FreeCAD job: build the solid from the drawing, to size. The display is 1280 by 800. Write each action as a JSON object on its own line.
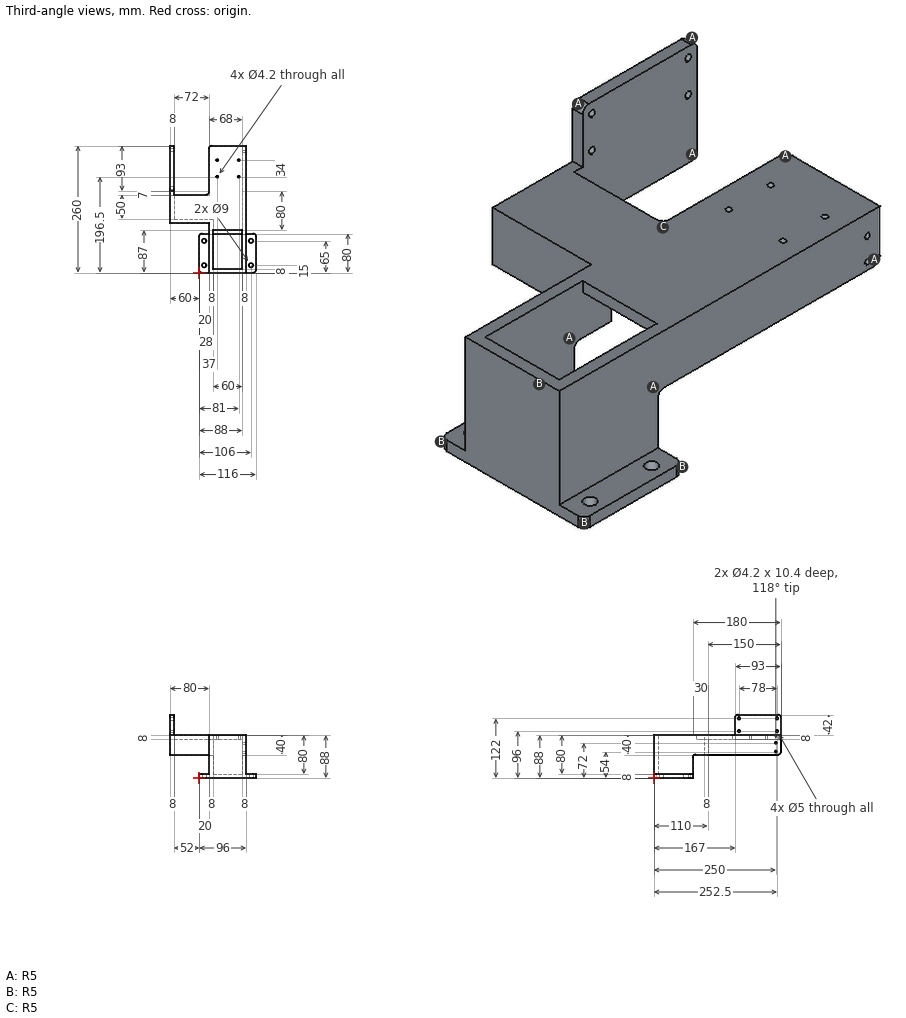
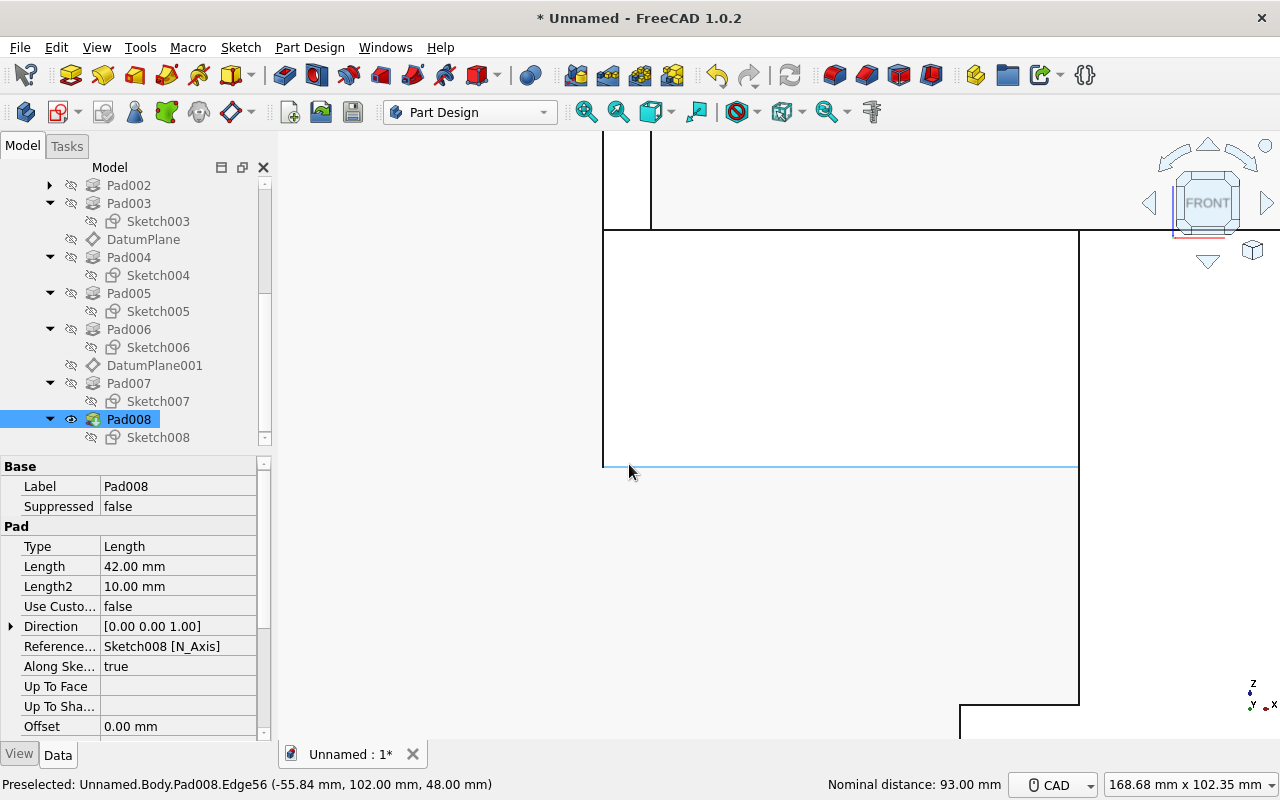
{"action": "left_click", "coordinate": [588, 112]}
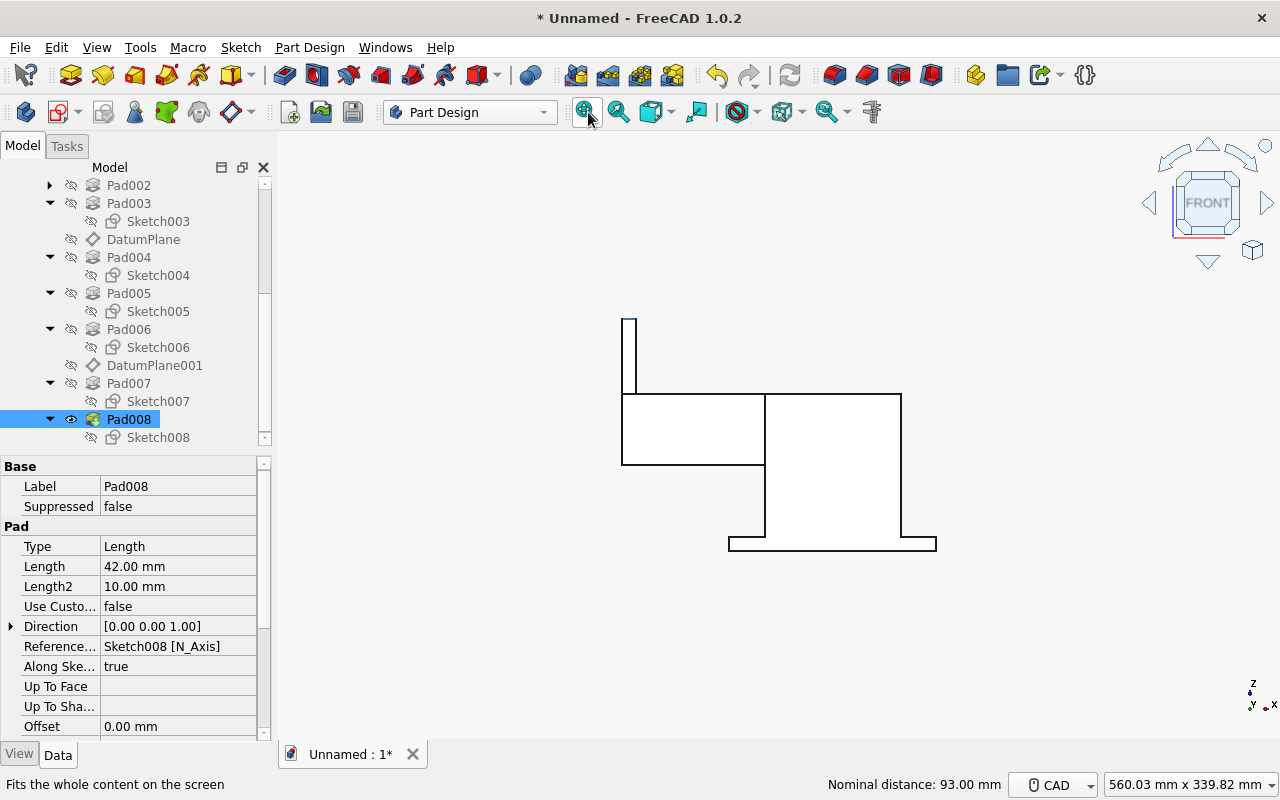
{"action": "key", "text": "3"}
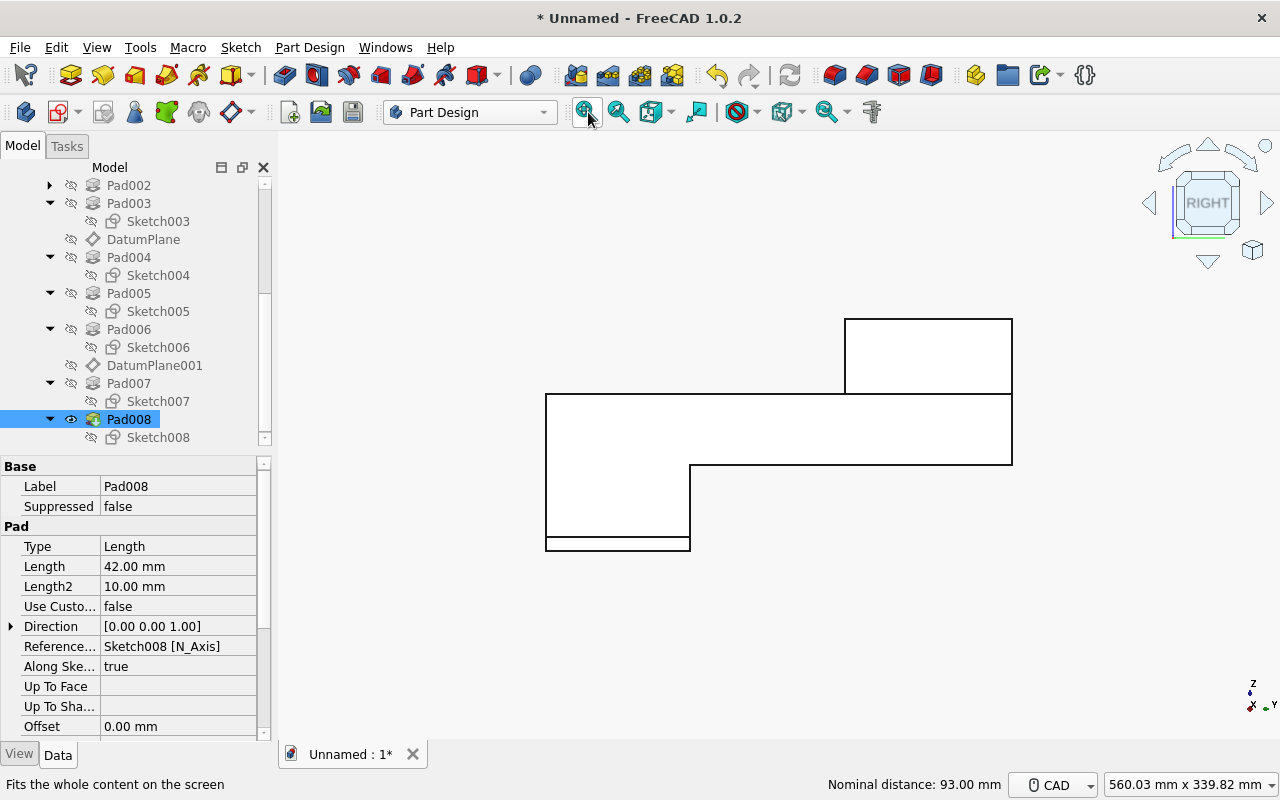
{"action": "scroll", "coordinate": [1012, 464], "scroll_direction": "up", "scroll_amount": 6}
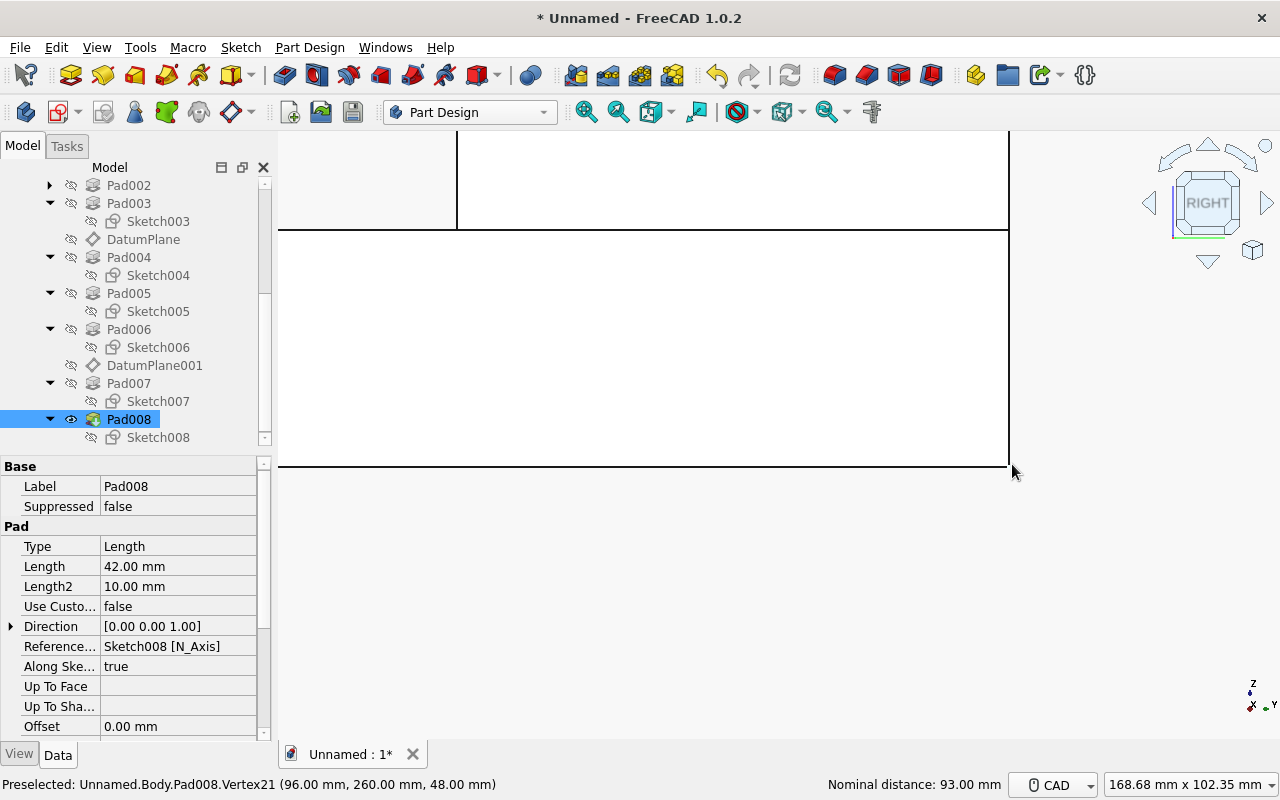
{"action": "left_click", "coordinate": [588, 112]}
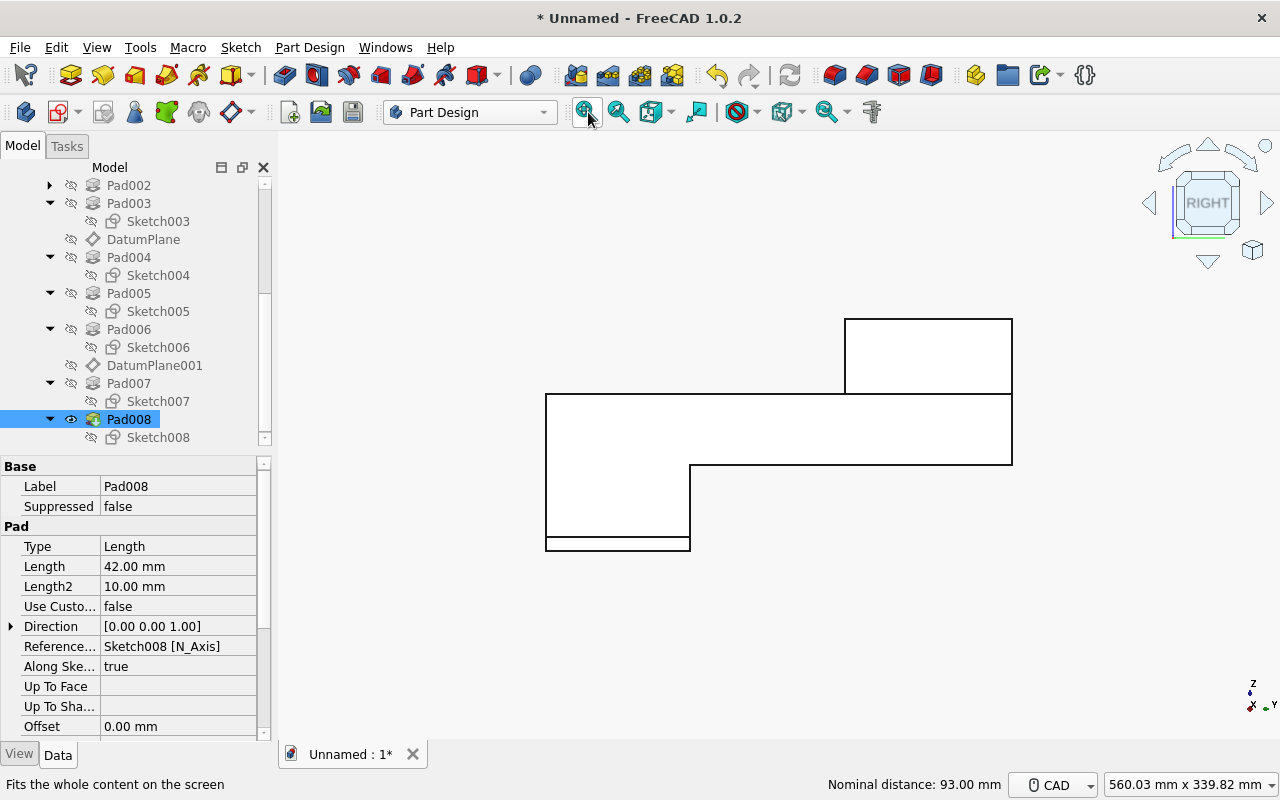
{"action": "key", "text": "5"}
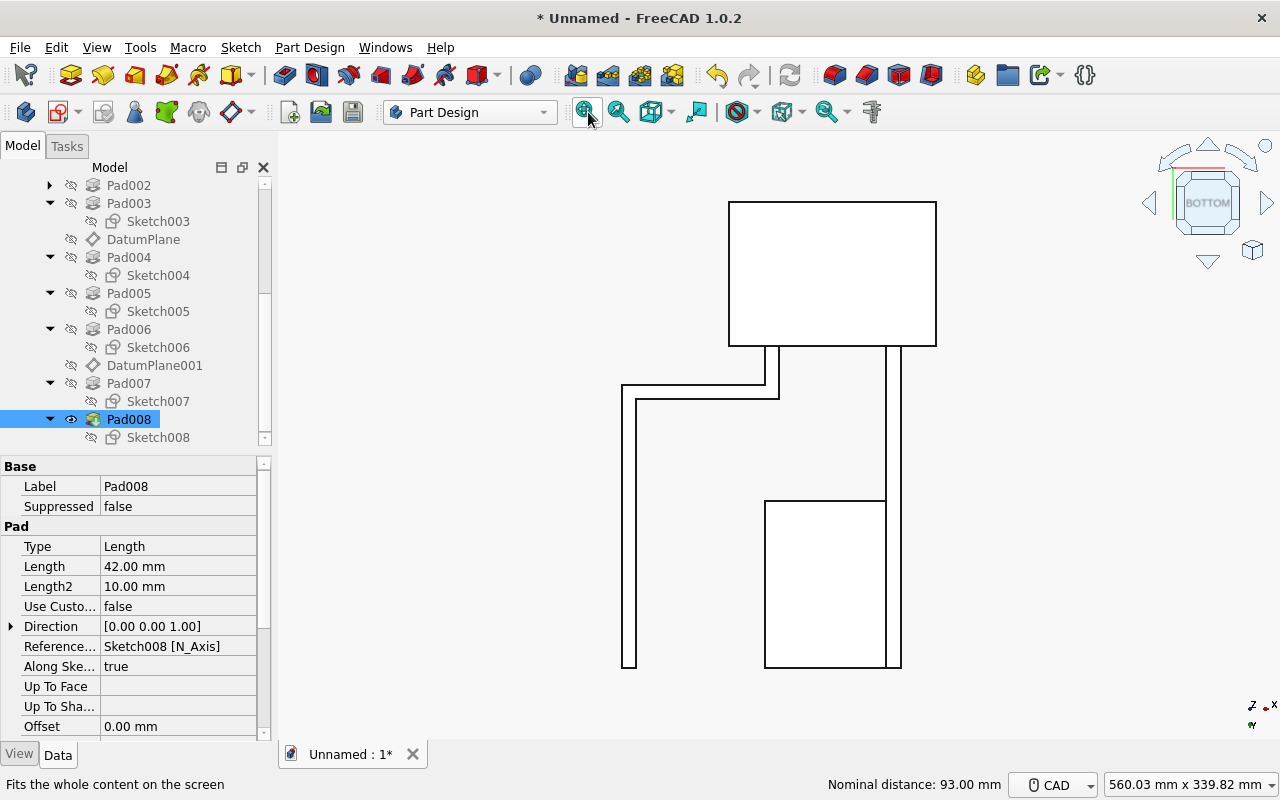
{"action": "left_click", "coordinate": [629, 667], "text": "ctrl"}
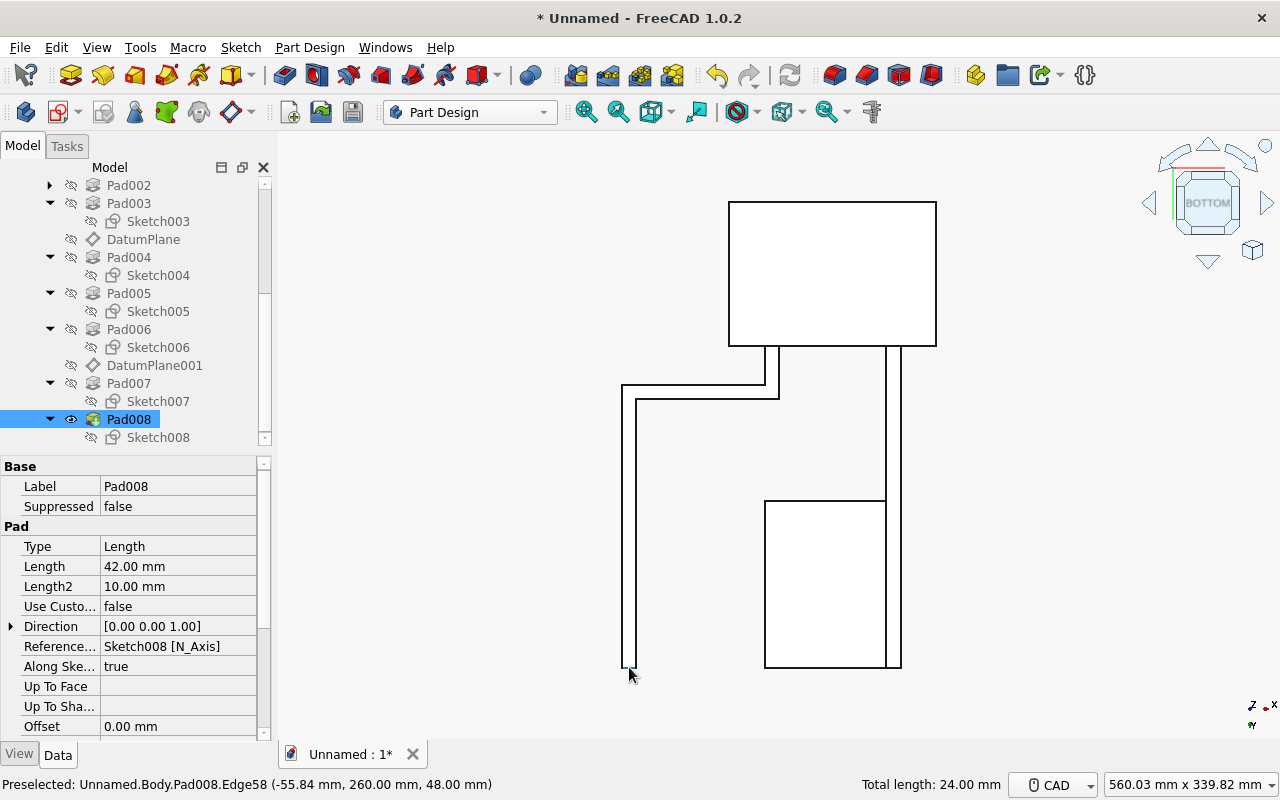
{"action": "left_click", "coordinate": [894, 667], "text": "ctrl"}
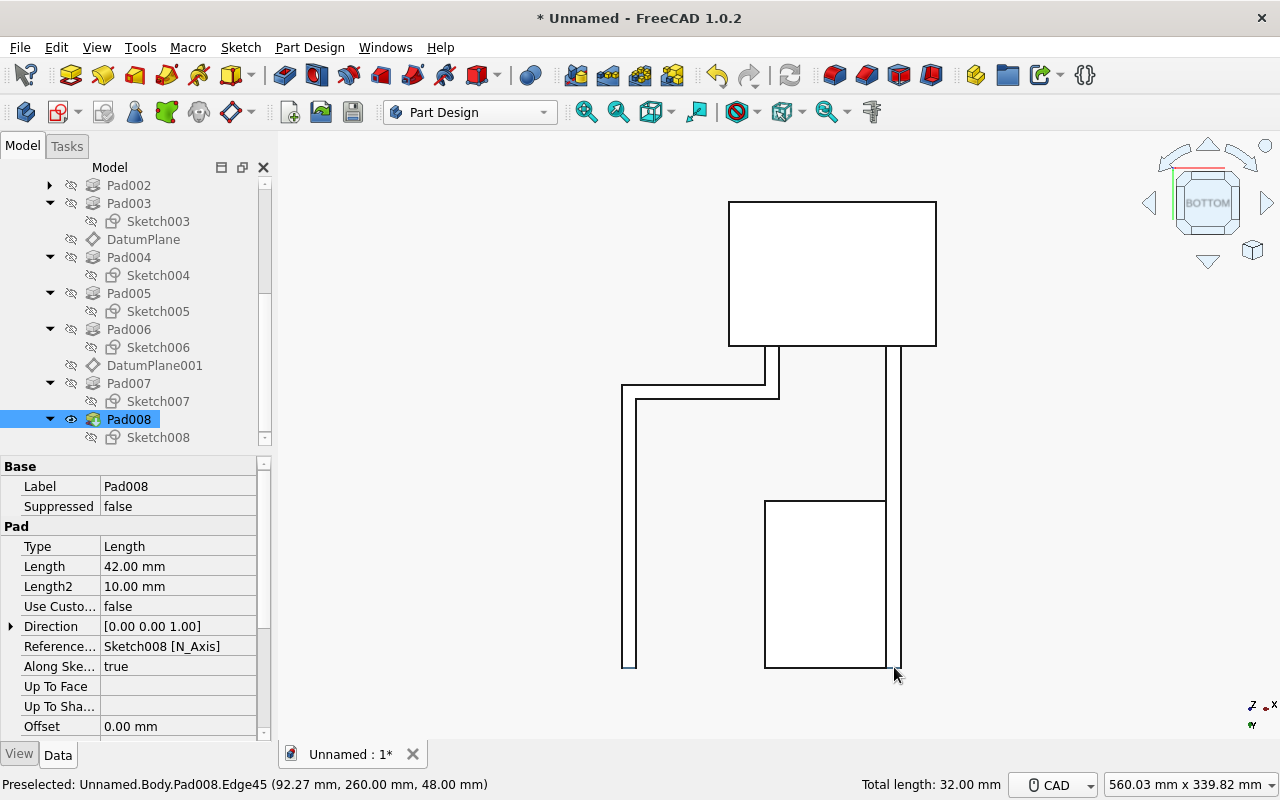
{"action": "scroll", "coordinate": [772, 345], "scroll_direction": "up", "scroll_amount": 6}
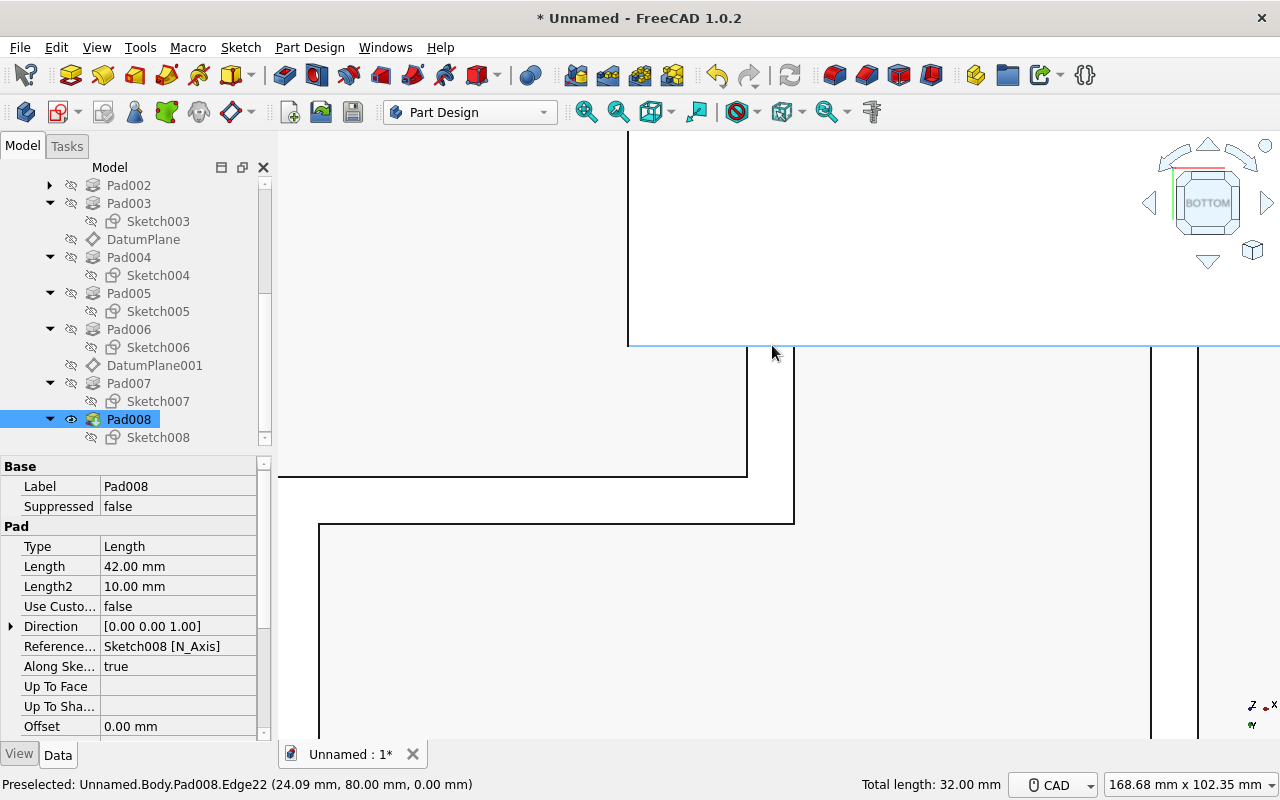
{"action": "left_click", "coordinate": [588, 112]}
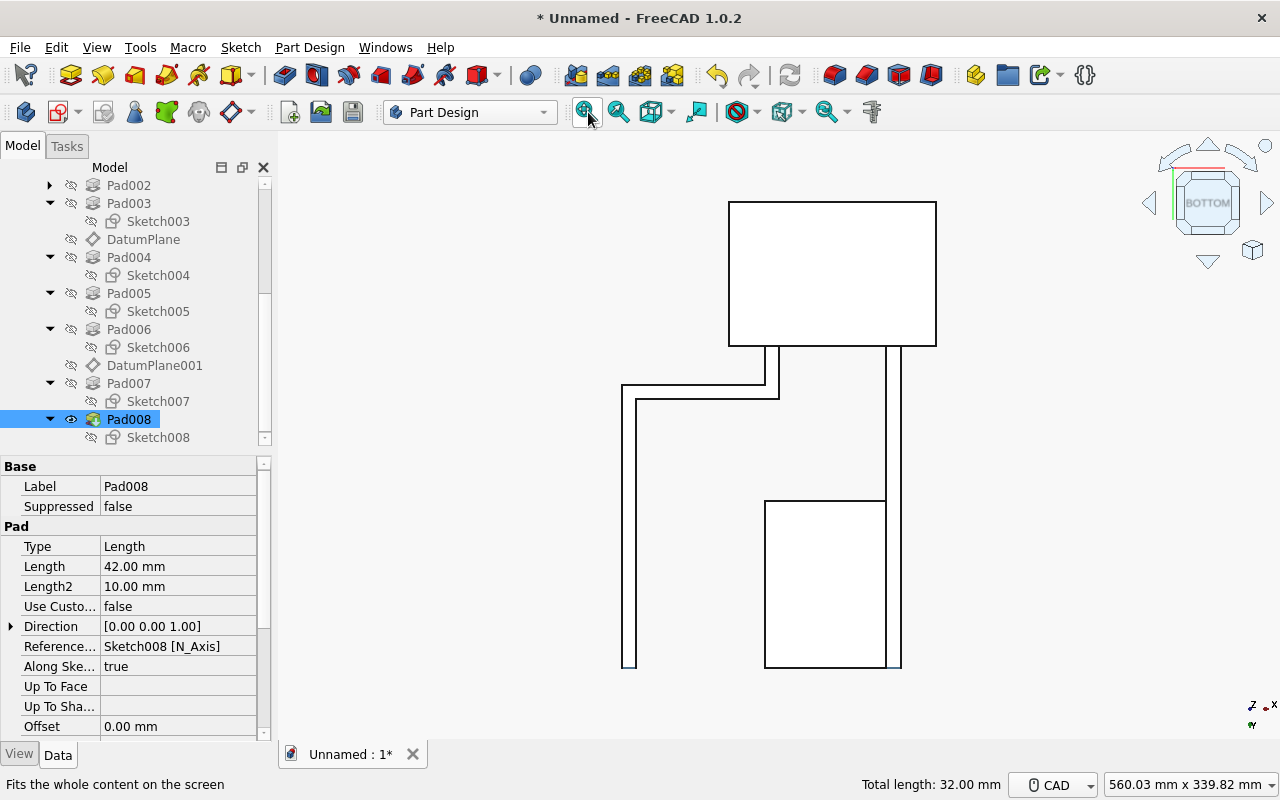
{"action": "key", "text": "4"}